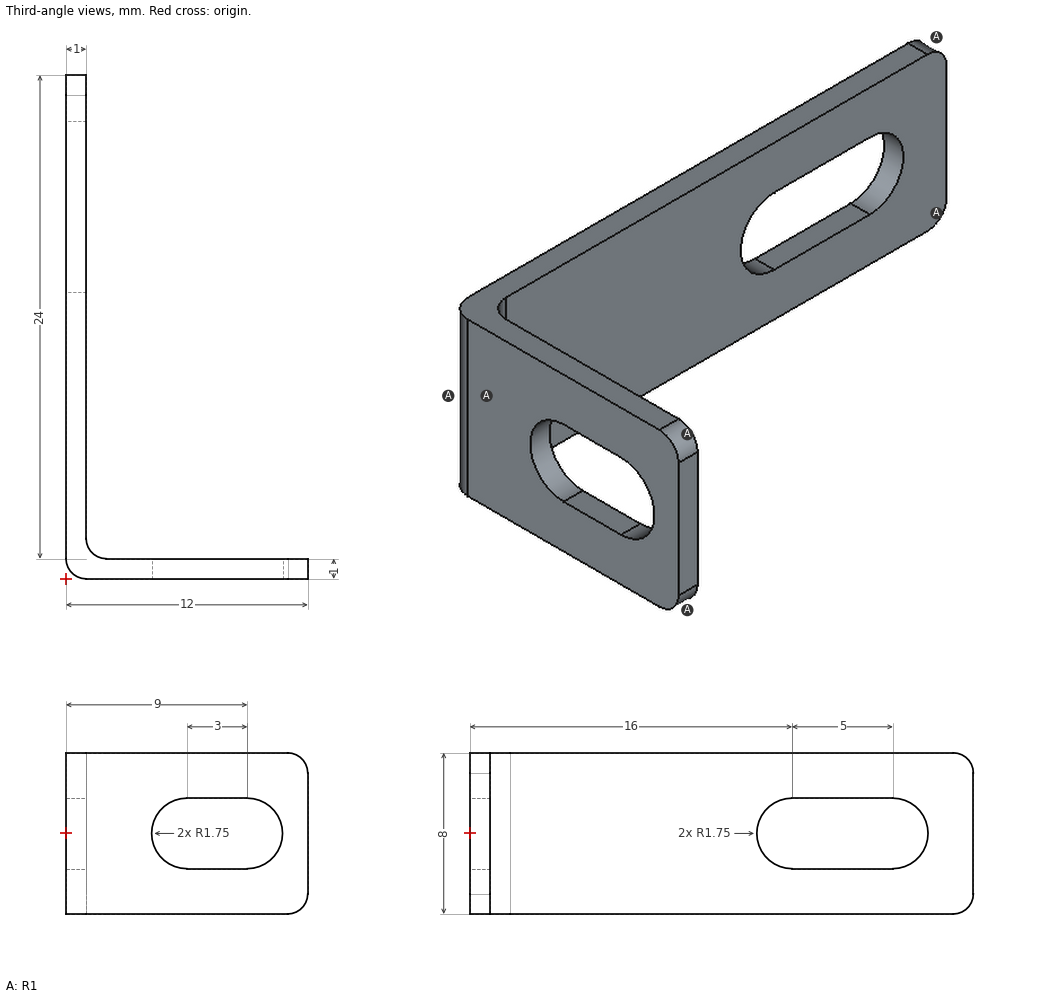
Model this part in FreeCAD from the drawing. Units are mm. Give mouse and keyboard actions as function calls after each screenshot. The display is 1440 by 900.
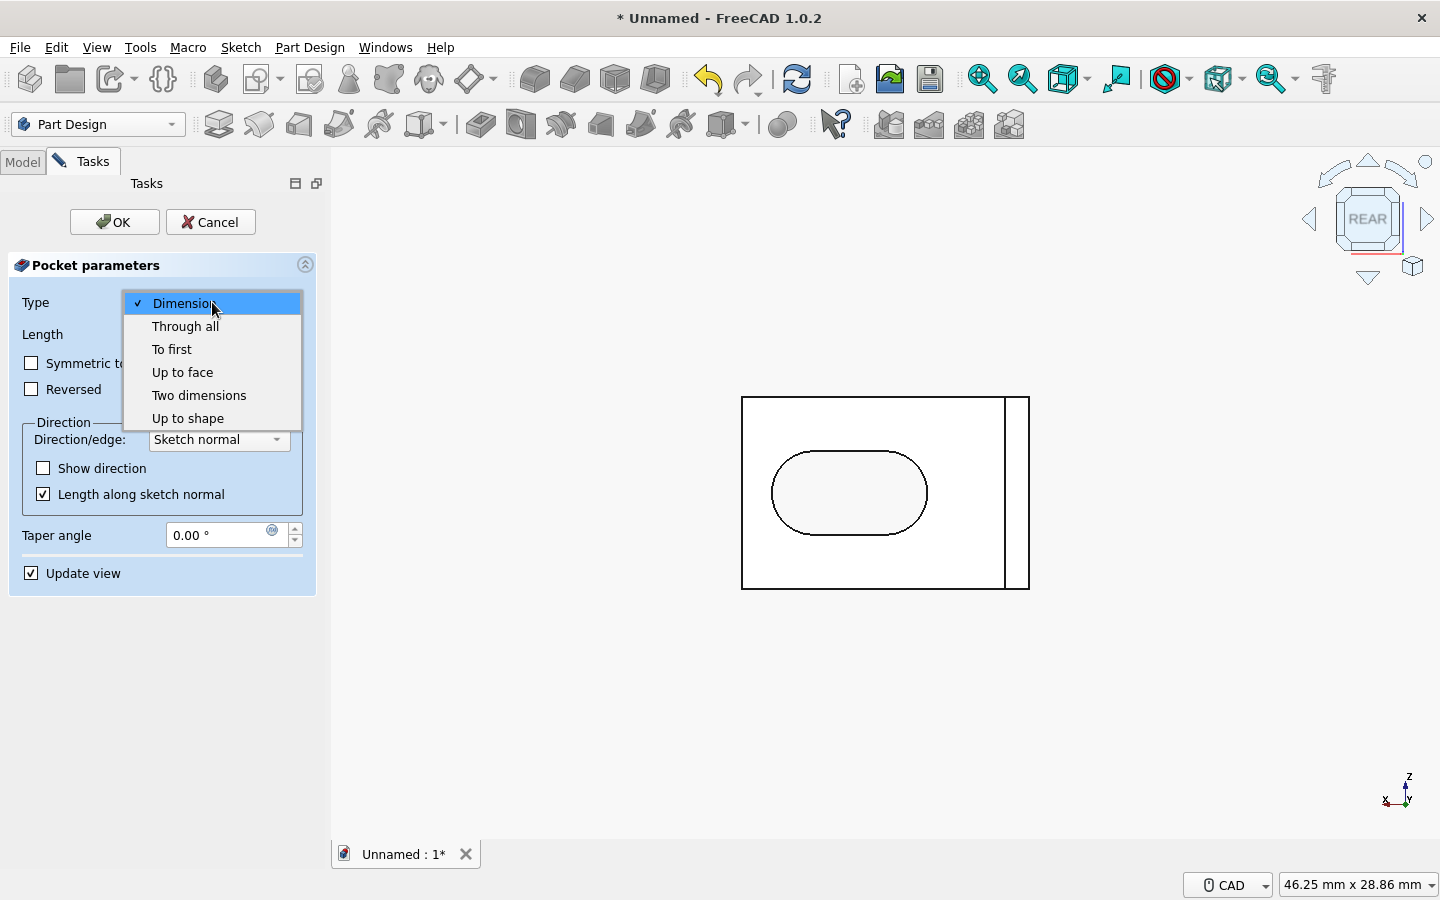
click(212, 326)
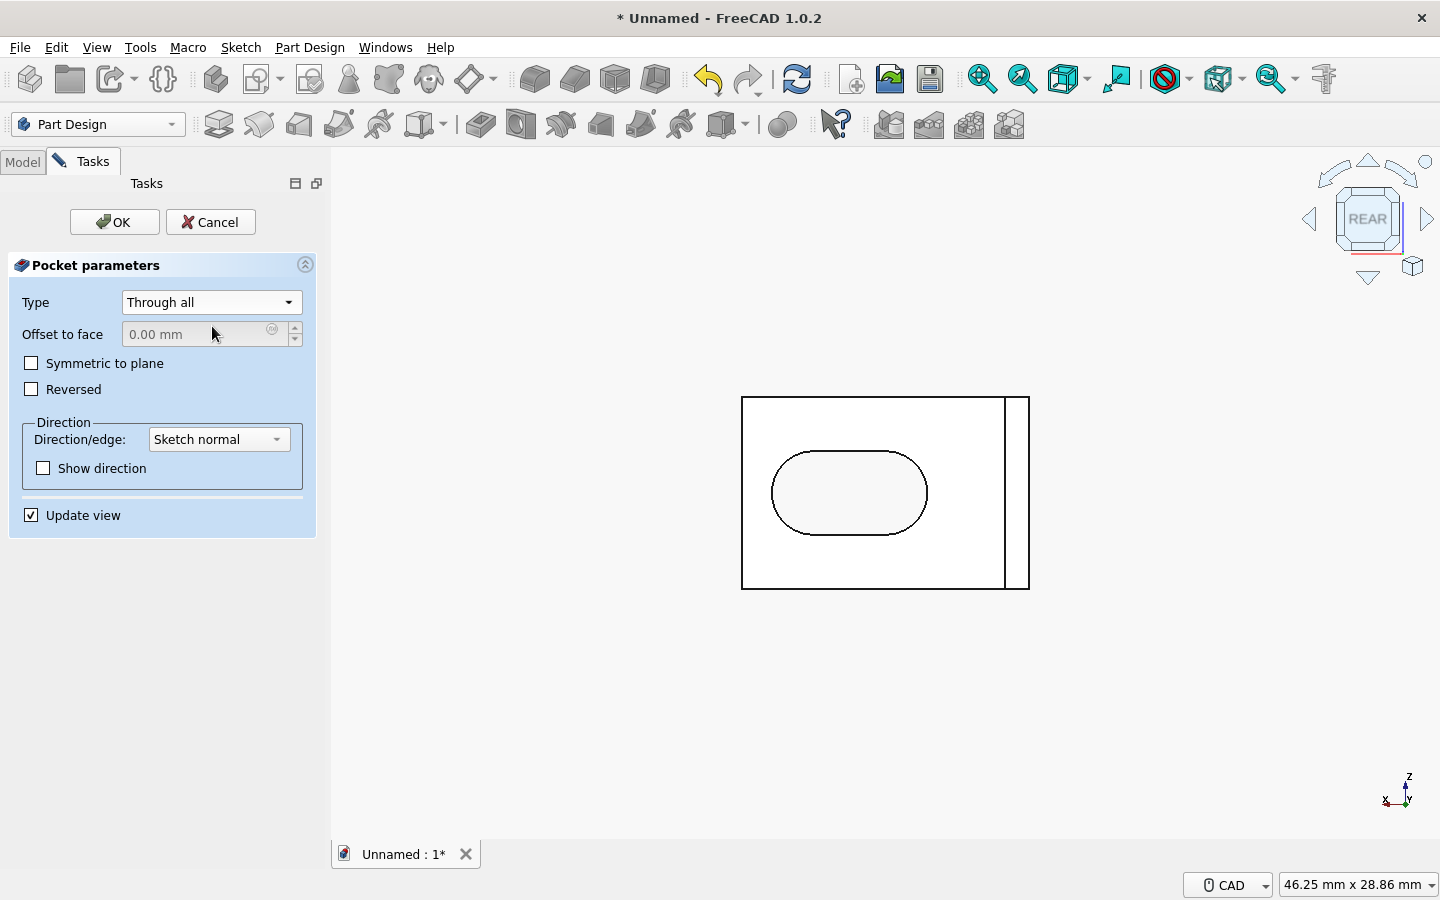
click(115, 222)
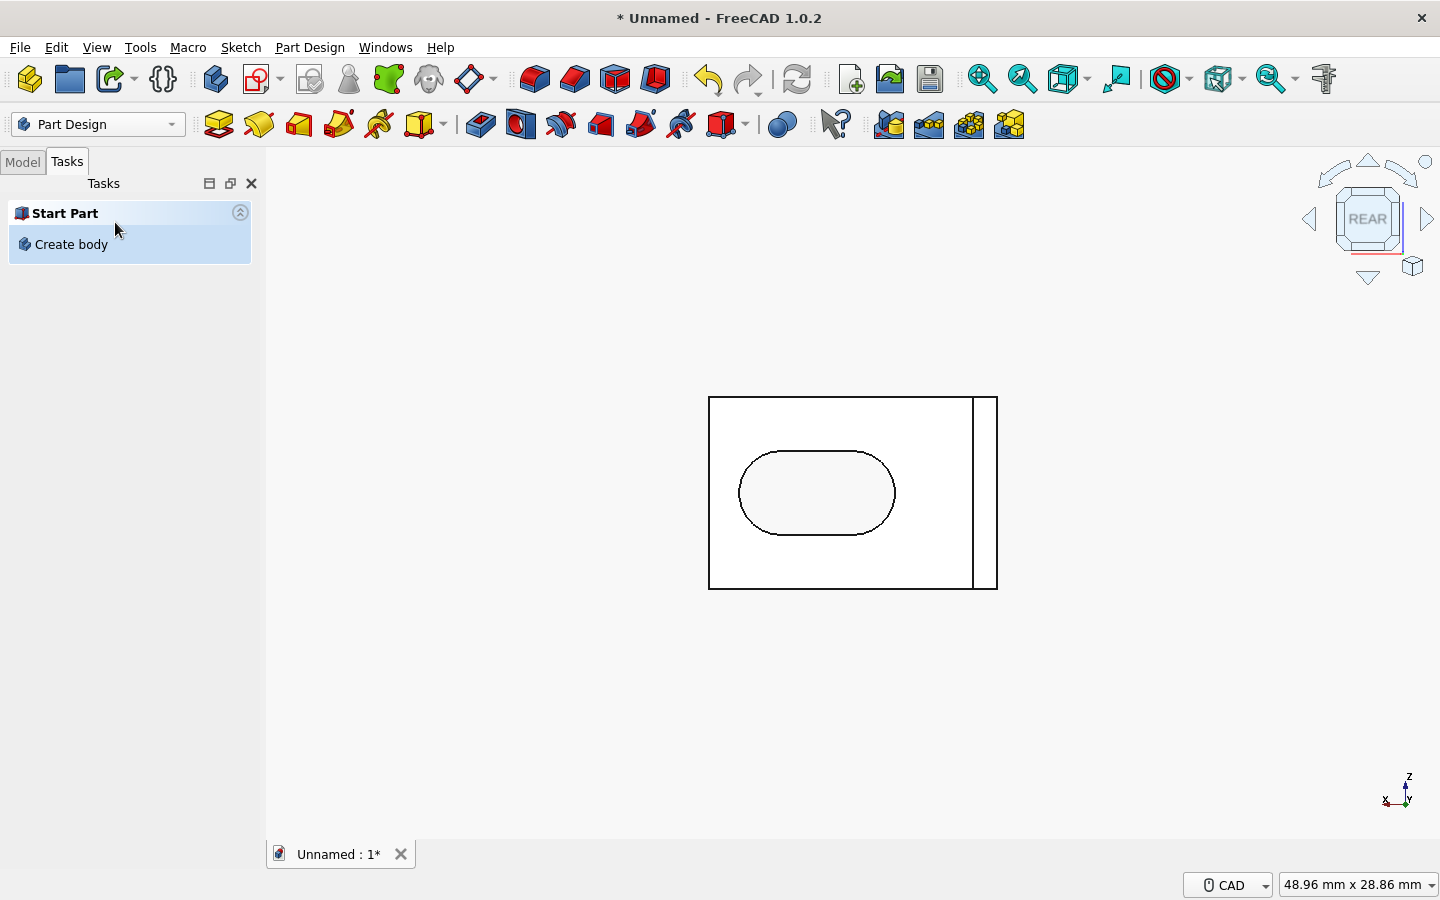
key(v)
key(f)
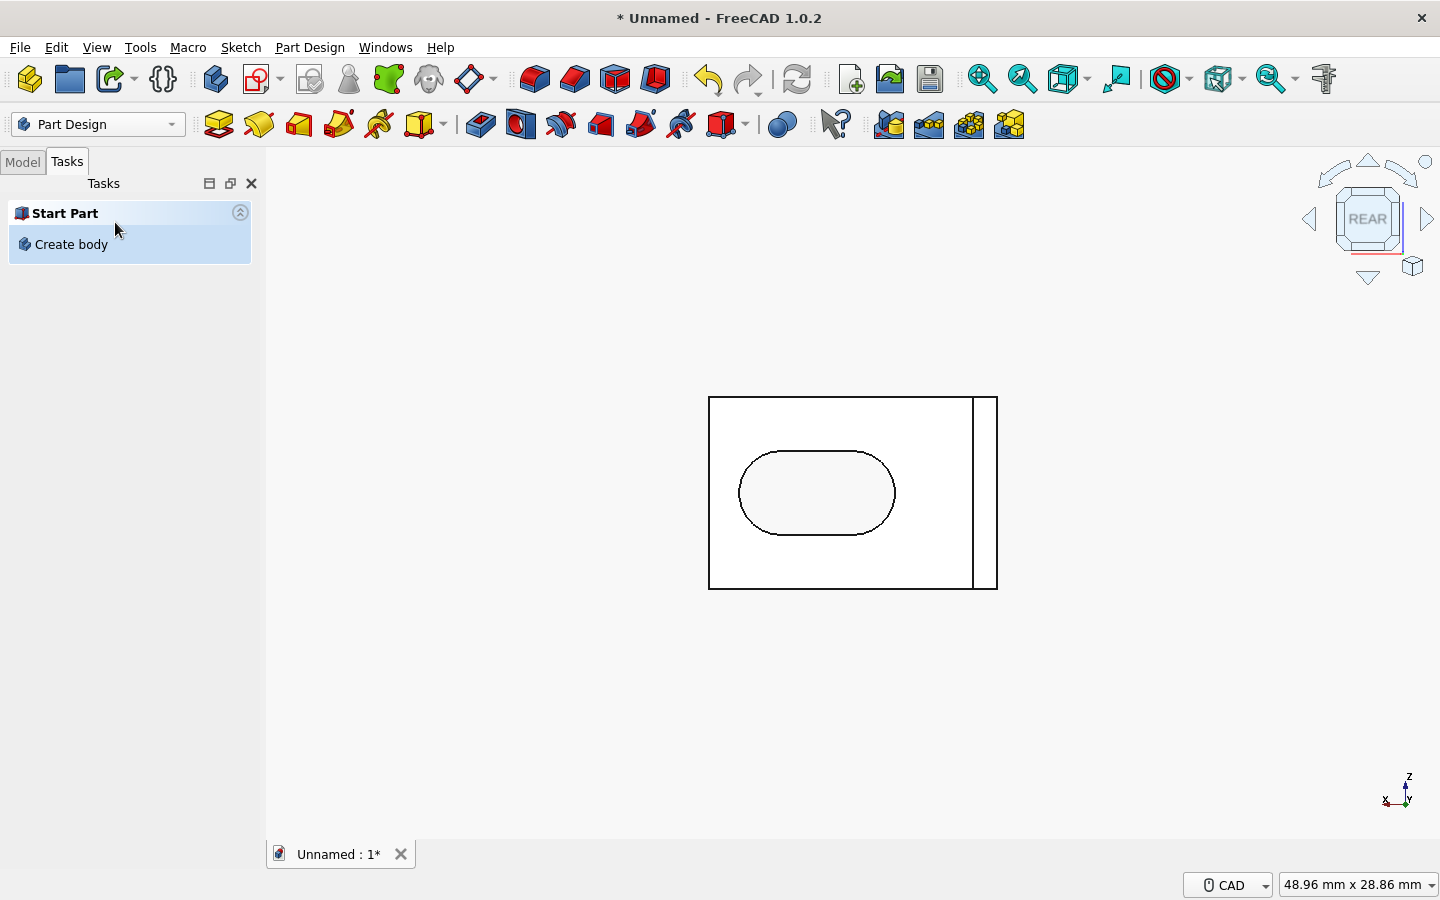
click(256, 80)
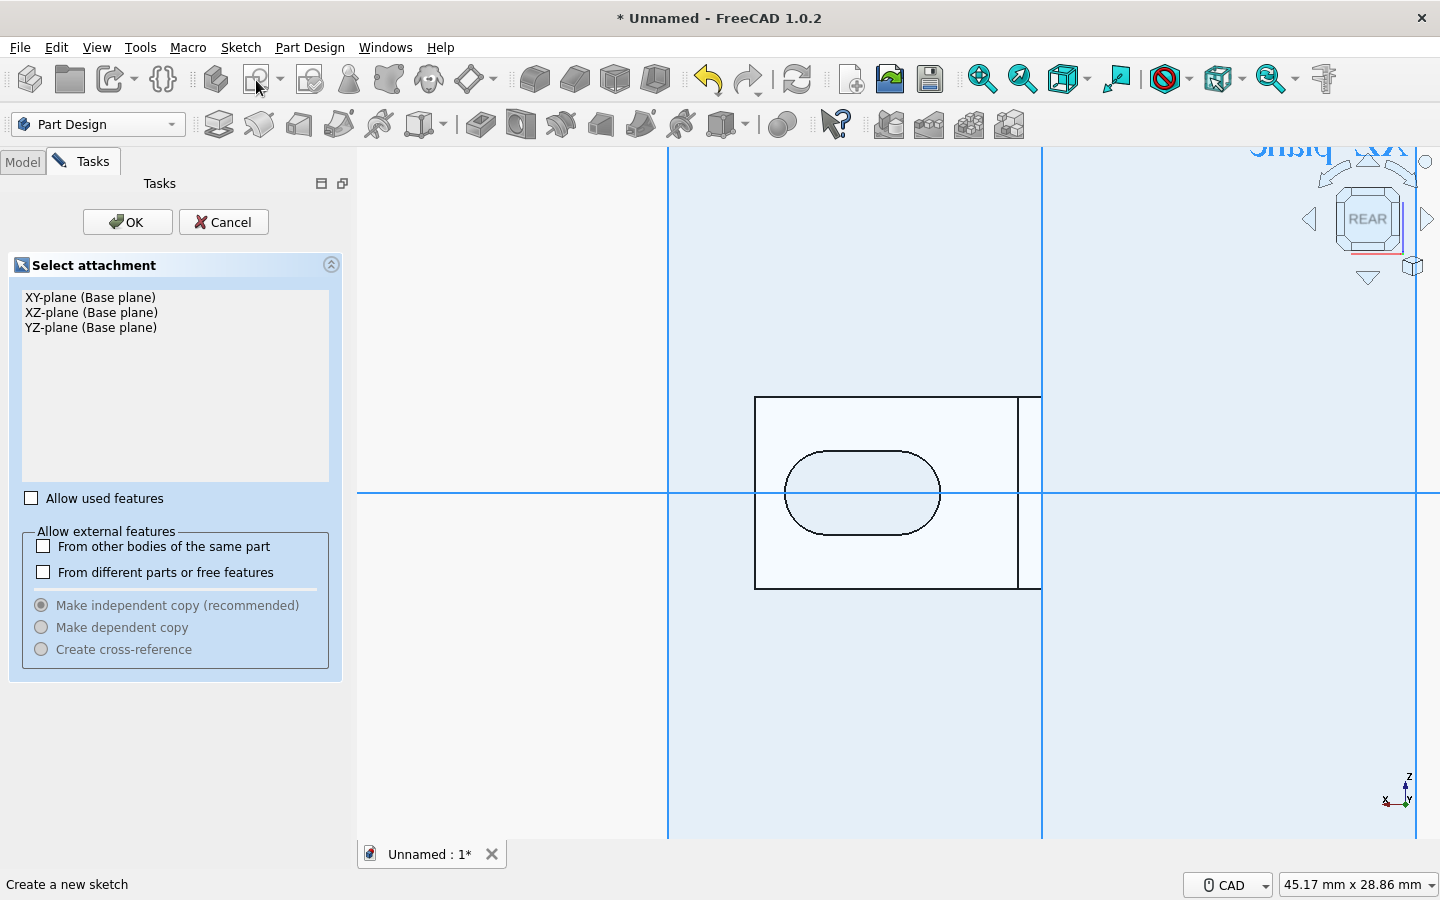
click(82, 328)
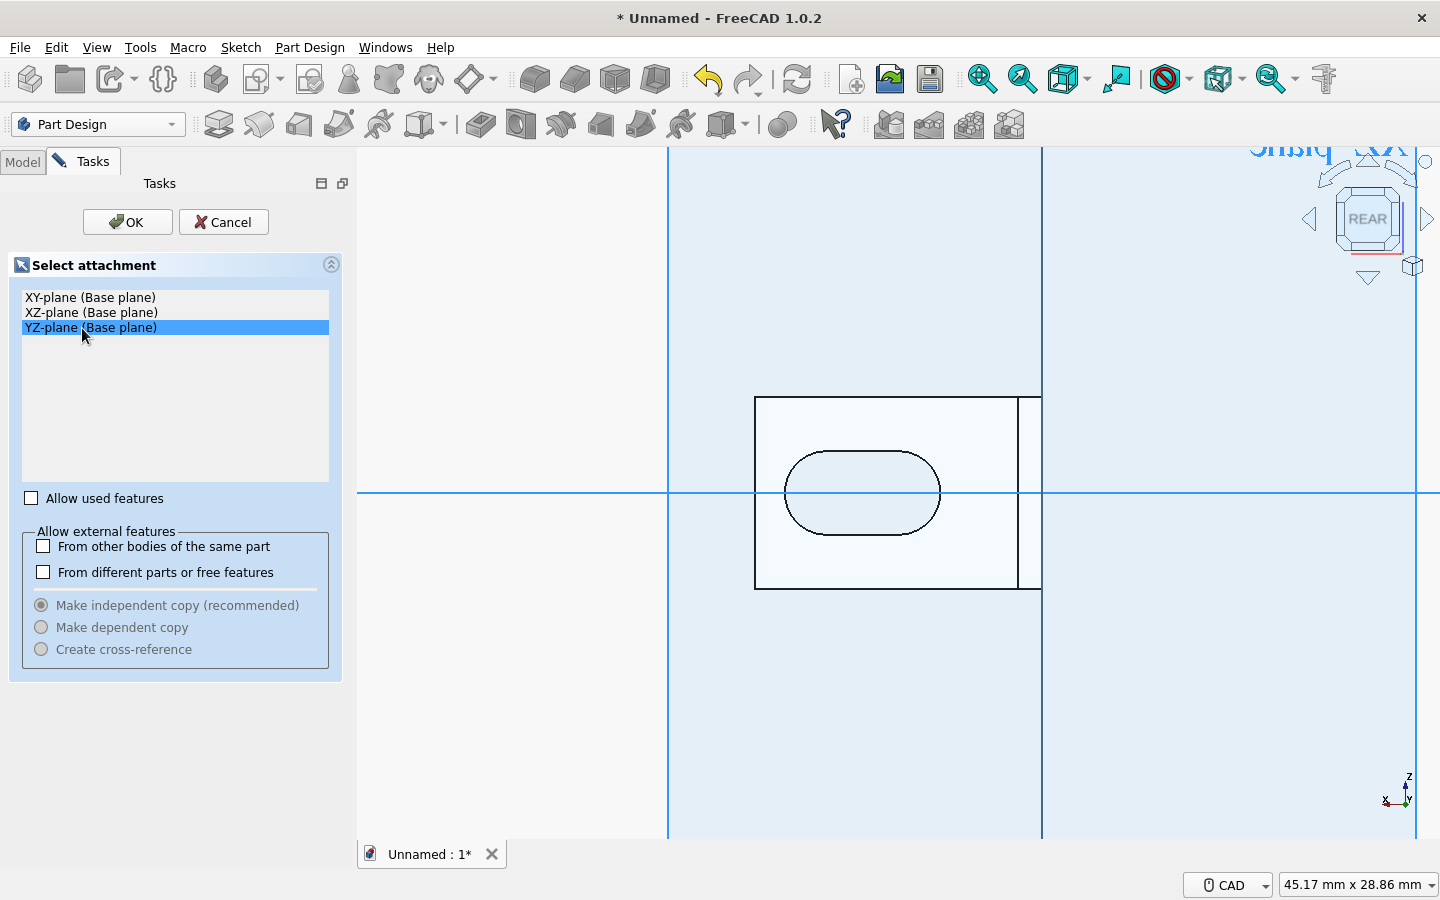
click(128, 222)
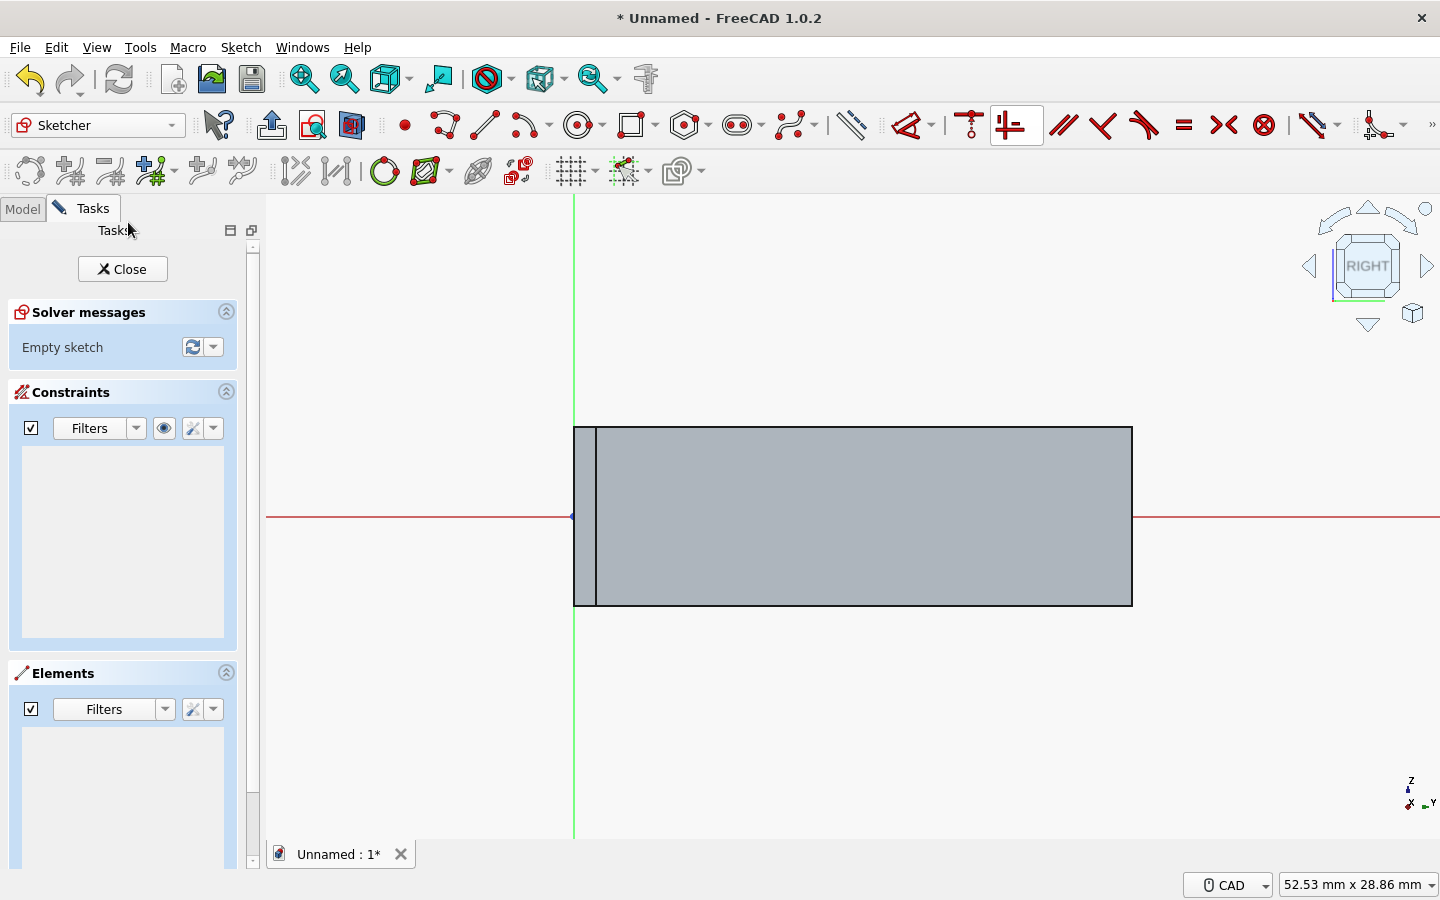
key(q)
key(s)